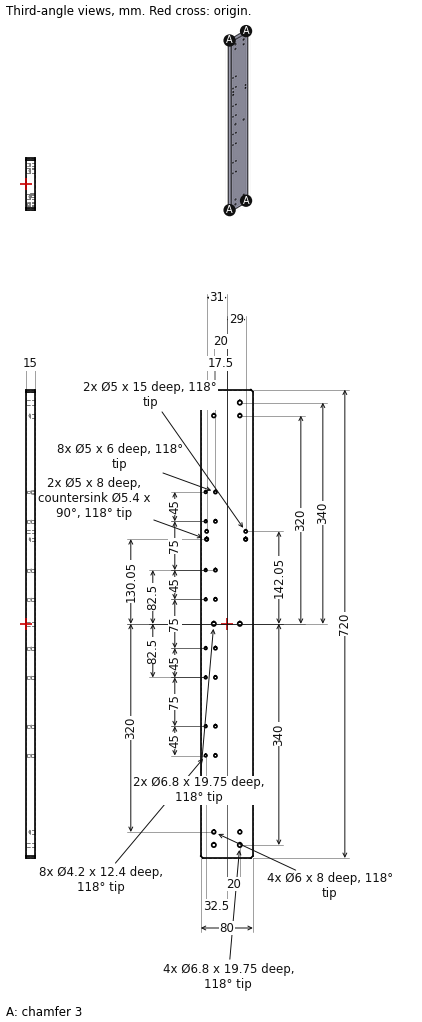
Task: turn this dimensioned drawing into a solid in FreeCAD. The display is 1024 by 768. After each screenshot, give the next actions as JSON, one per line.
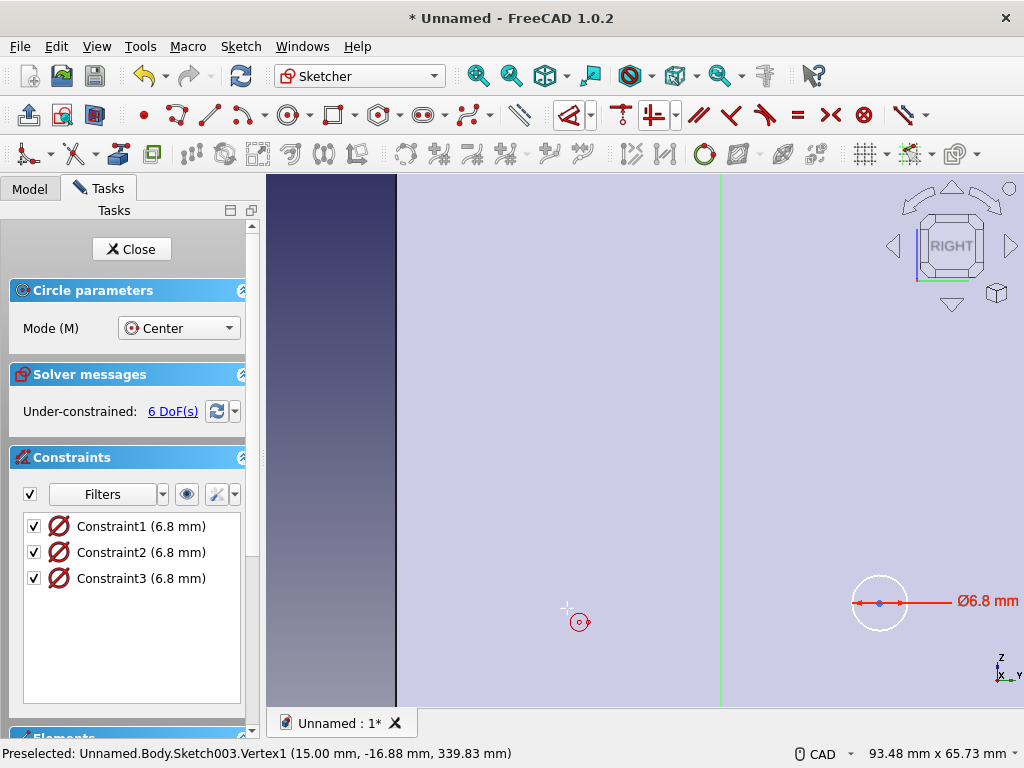
{"action": "scroll", "coordinate": [567, 609], "scroll_direction": "down", "scroll_amount": 14}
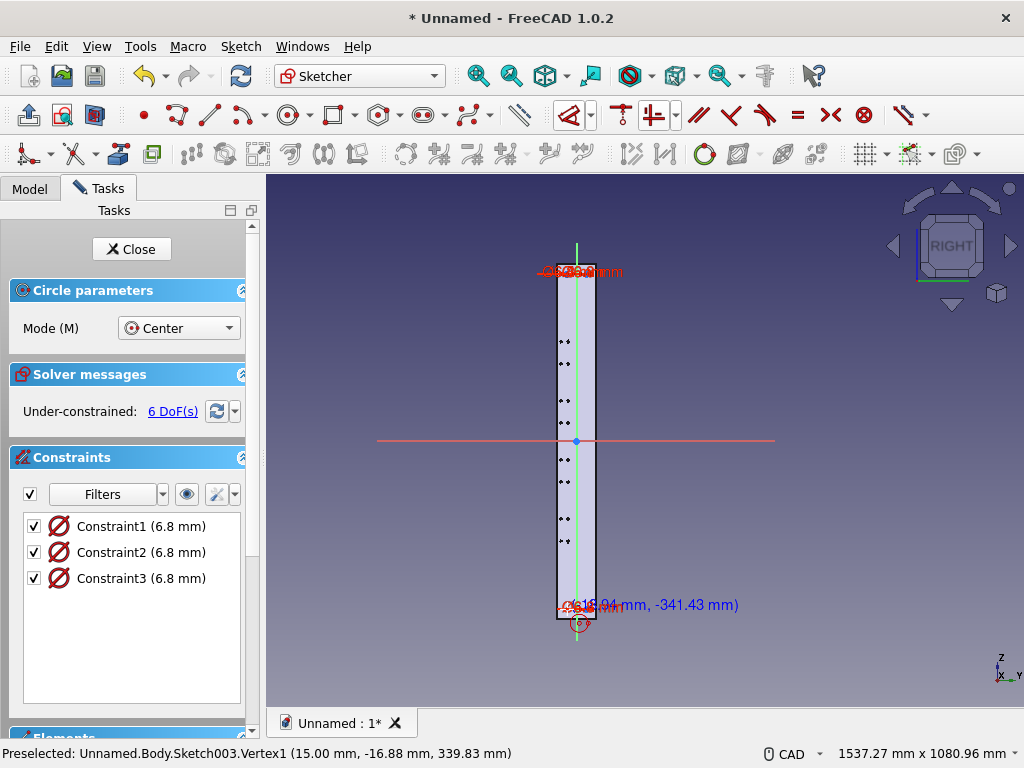
{"action": "scroll", "coordinate": [567, 609], "scroll_direction": "up", "scroll_amount": 3}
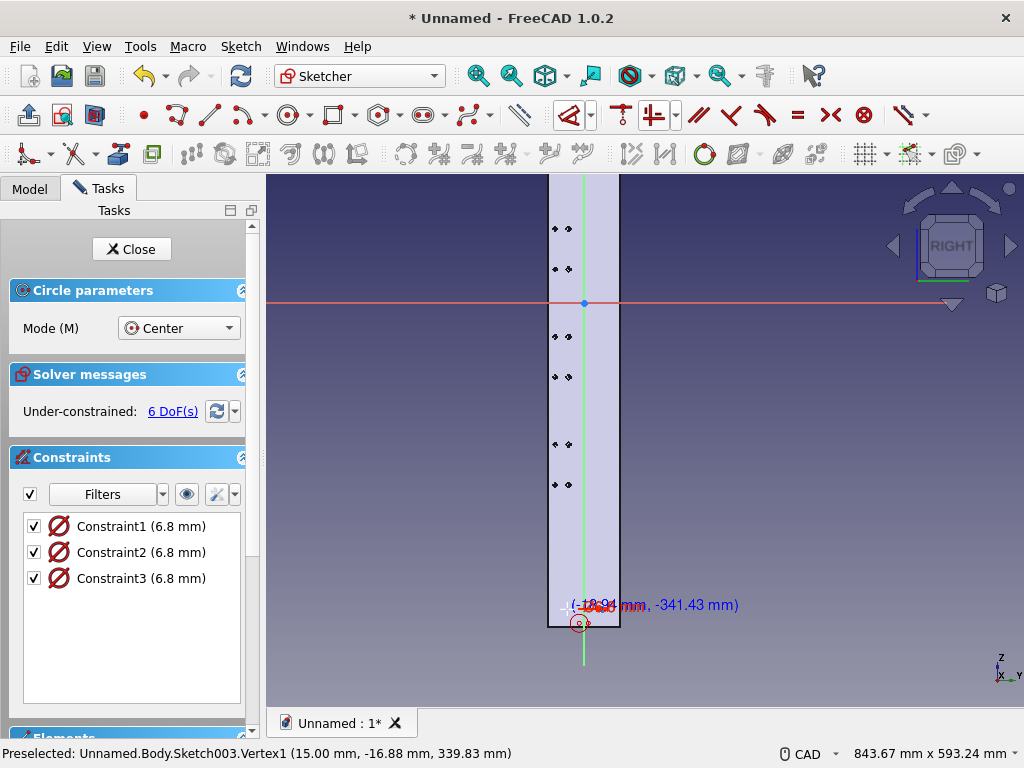
{"action": "left_click", "coordinate": [566, 609]}
{"action": "mouse_move", "coordinate": [569, 606]}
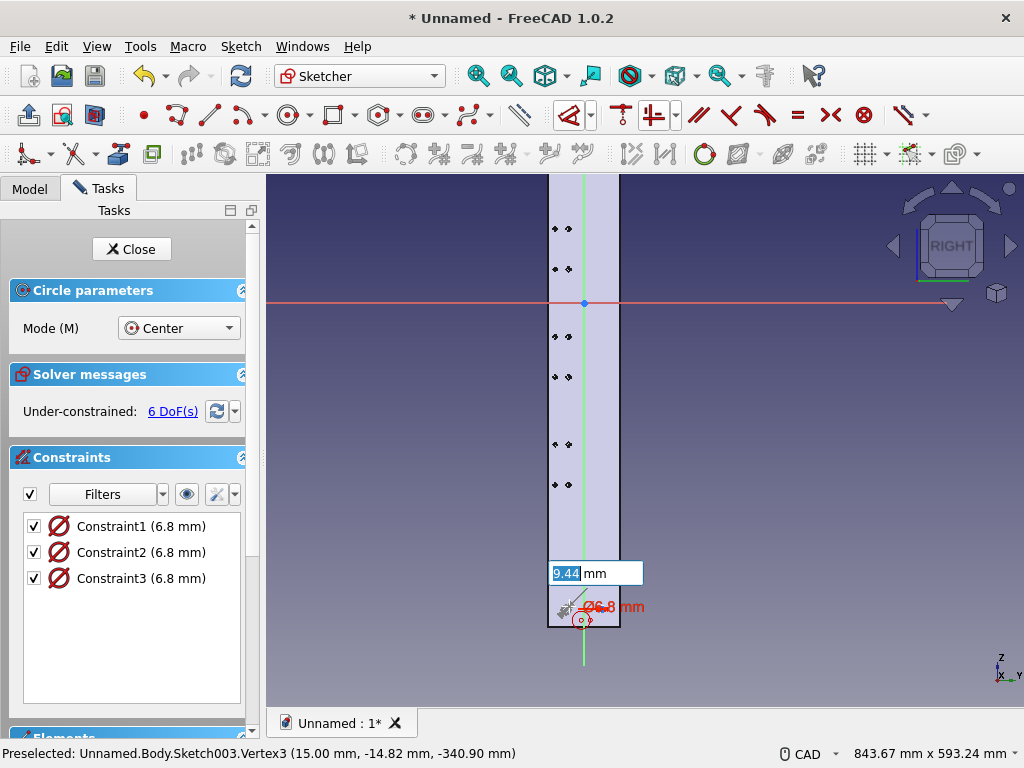
{"action": "type", "text": "6.8"}
{"action": "key", "text": "Return"}
{"action": "key", "text": "Escape"}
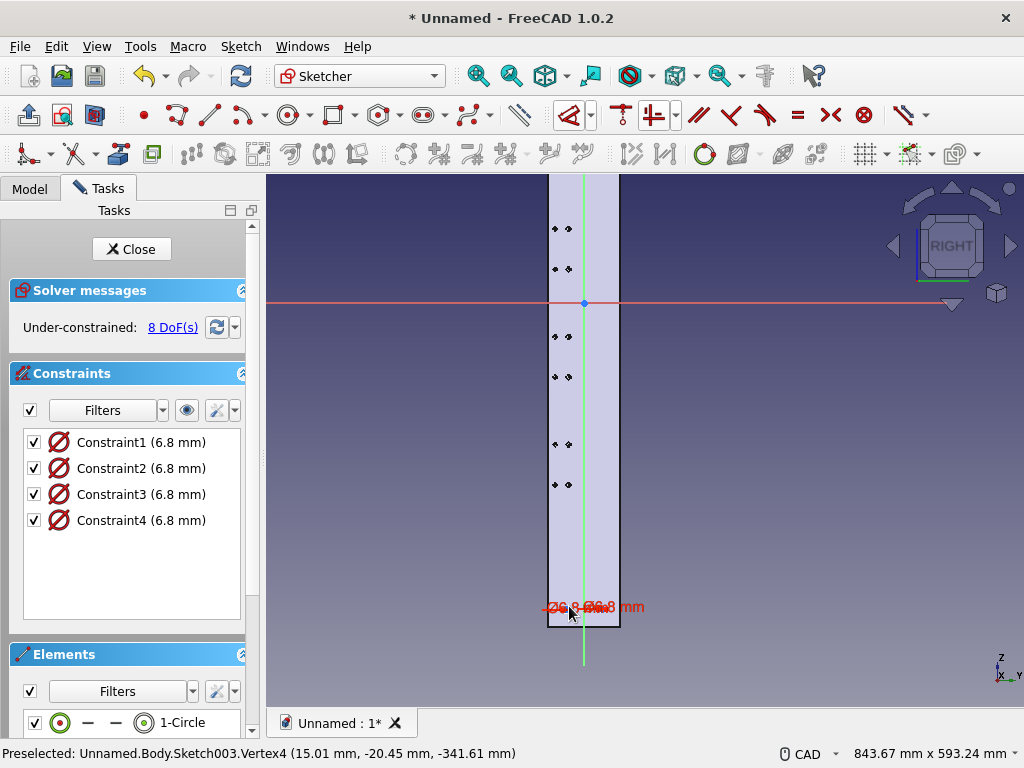
{"action": "left_click", "coordinate": [602, 609]}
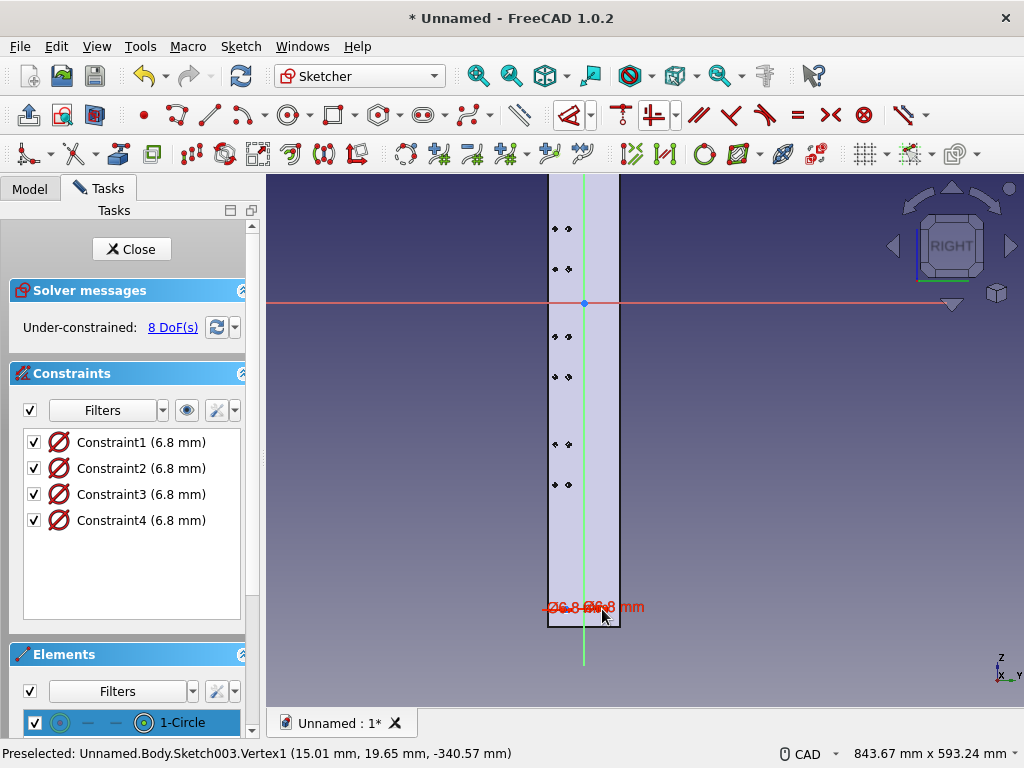
{"action": "scroll", "coordinate": [567, 608], "scroll_direction": "down", "scroll_amount": 3}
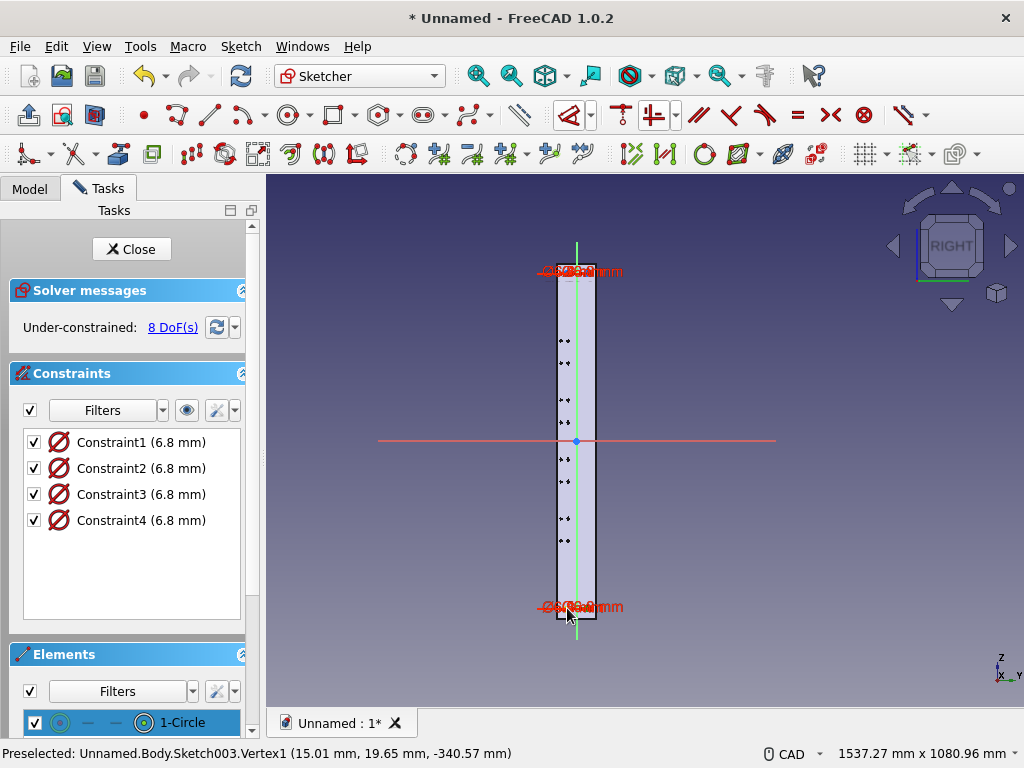
{"action": "left_click", "coordinate": [586, 274]}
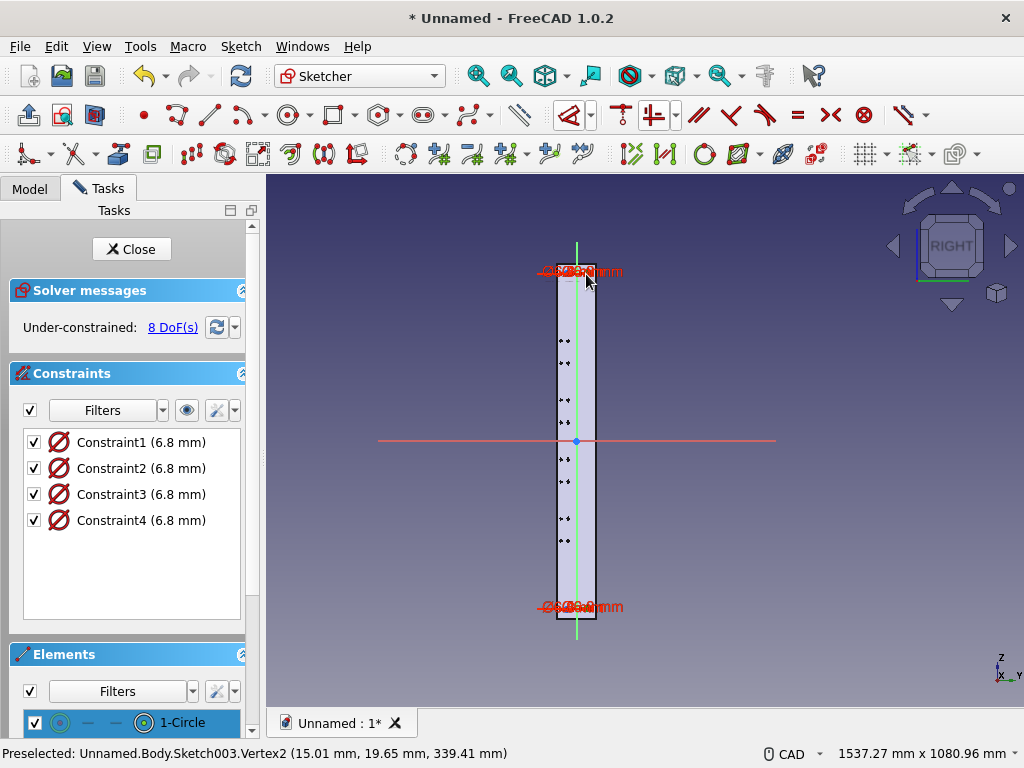
{"action": "left_click", "coordinate": [676, 116]}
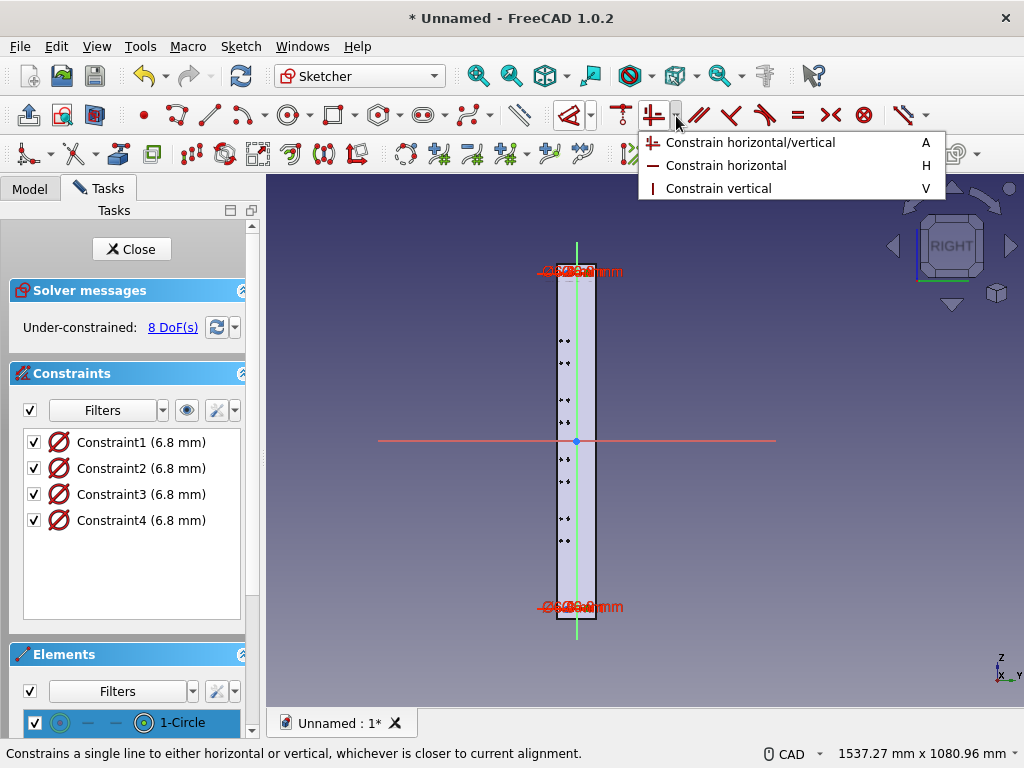
{"action": "left_click", "coordinate": [792, 188]}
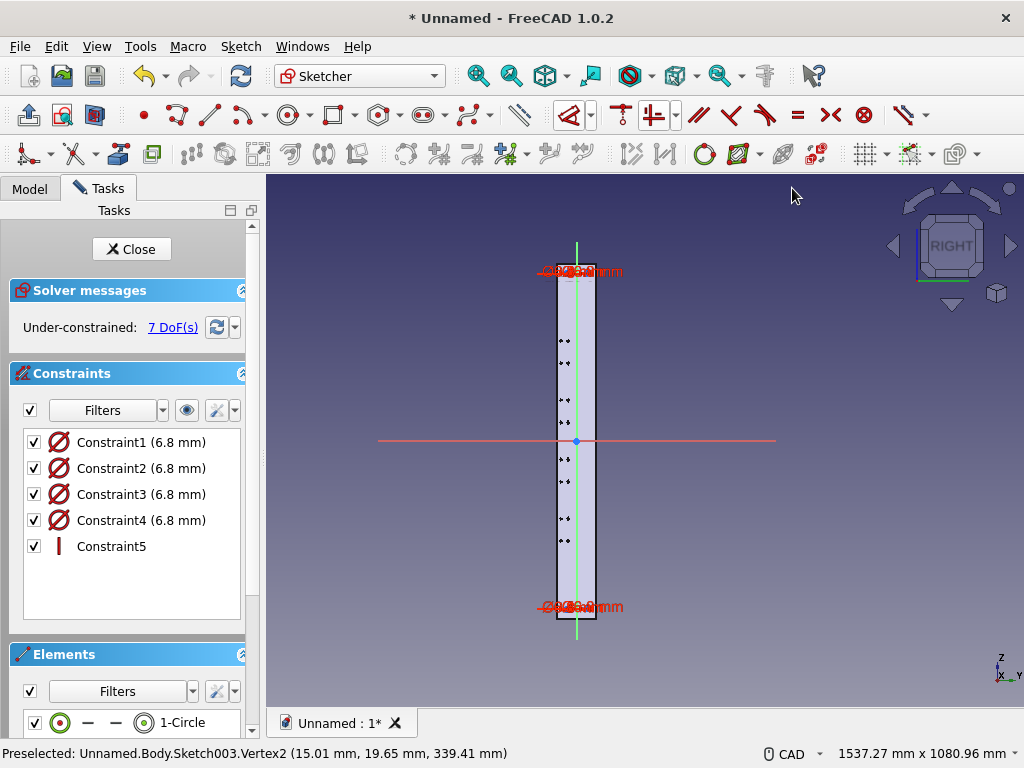
{"action": "left_click", "coordinate": [586, 274]}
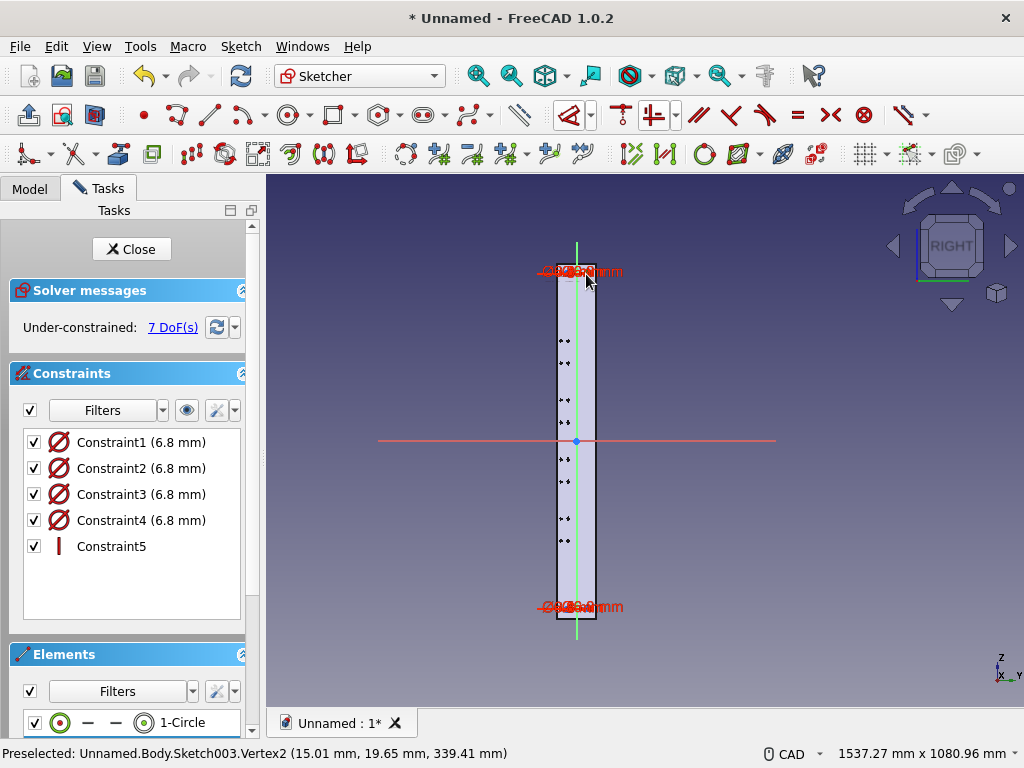
{"action": "scroll", "coordinate": [567, 274], "scroll_direction": "up", "scroll_amount": 4}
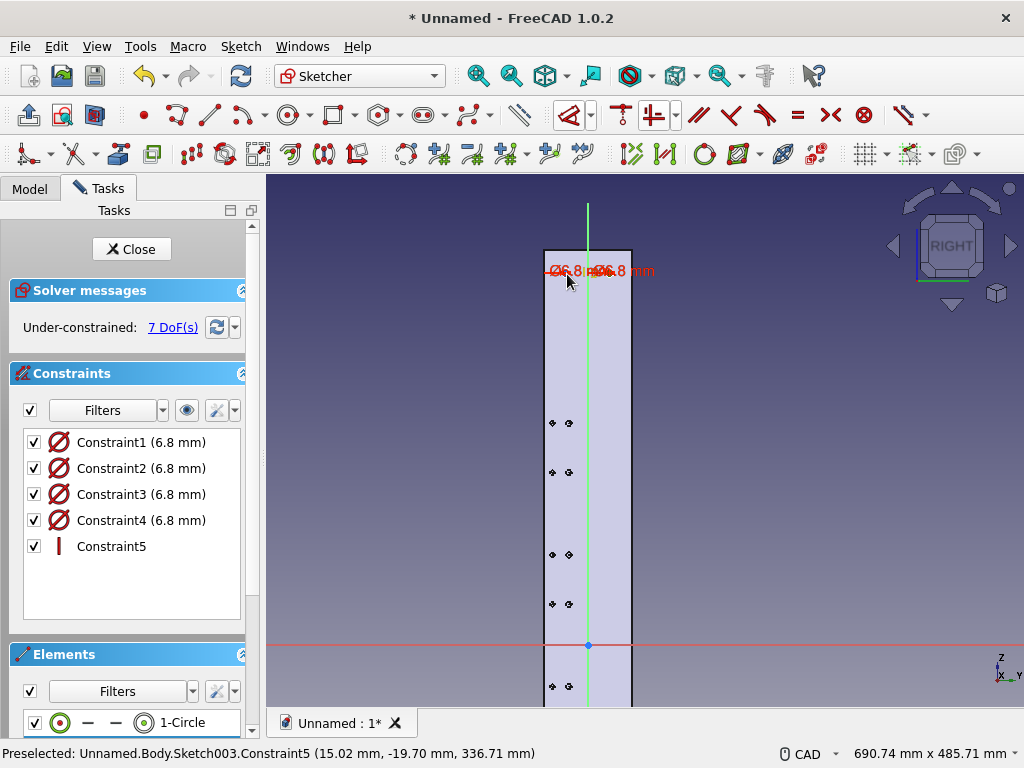
{"action": "left_click", "coordinate": [566, 273]}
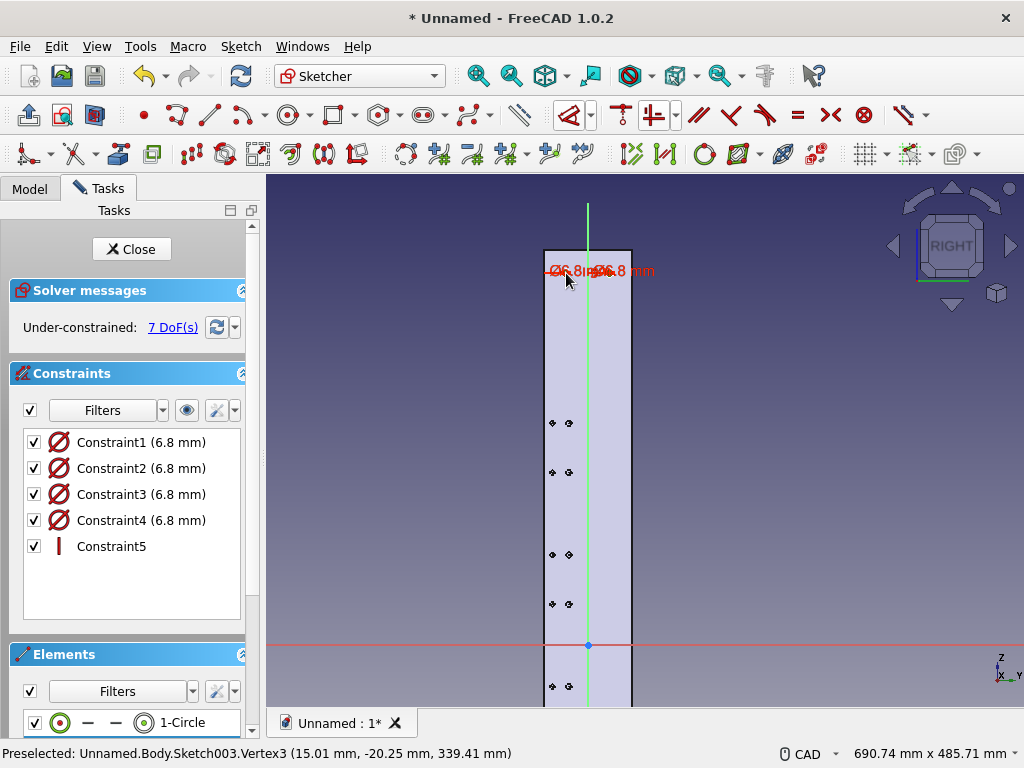
{"action": "key", "text": "h"}